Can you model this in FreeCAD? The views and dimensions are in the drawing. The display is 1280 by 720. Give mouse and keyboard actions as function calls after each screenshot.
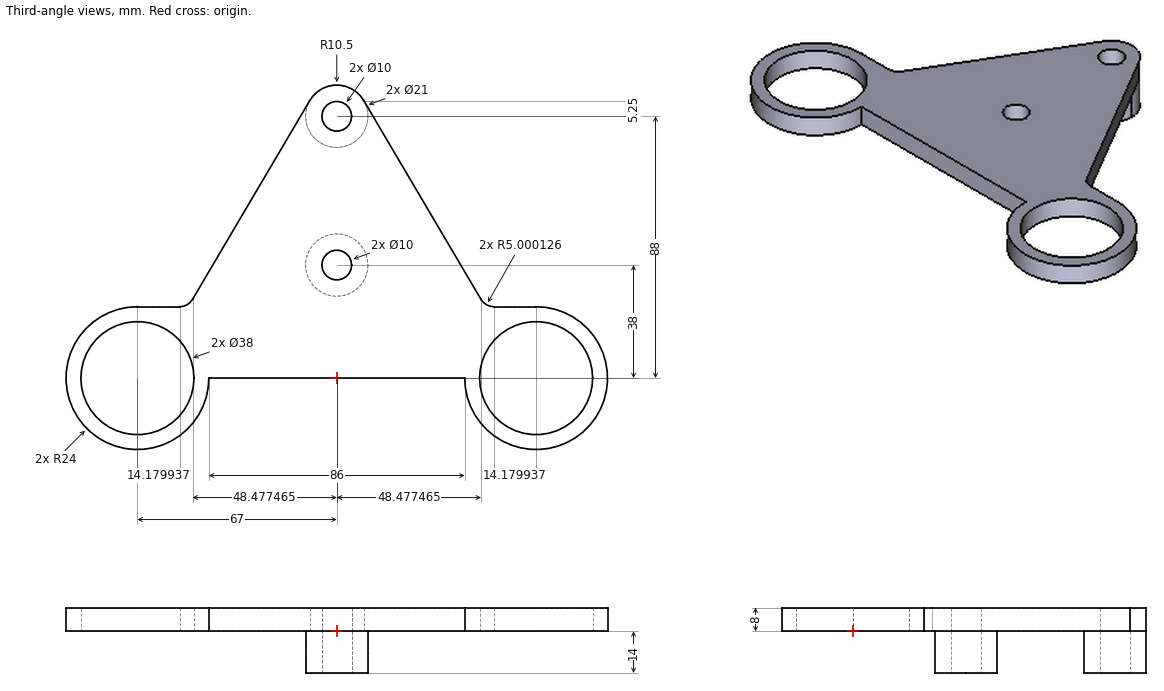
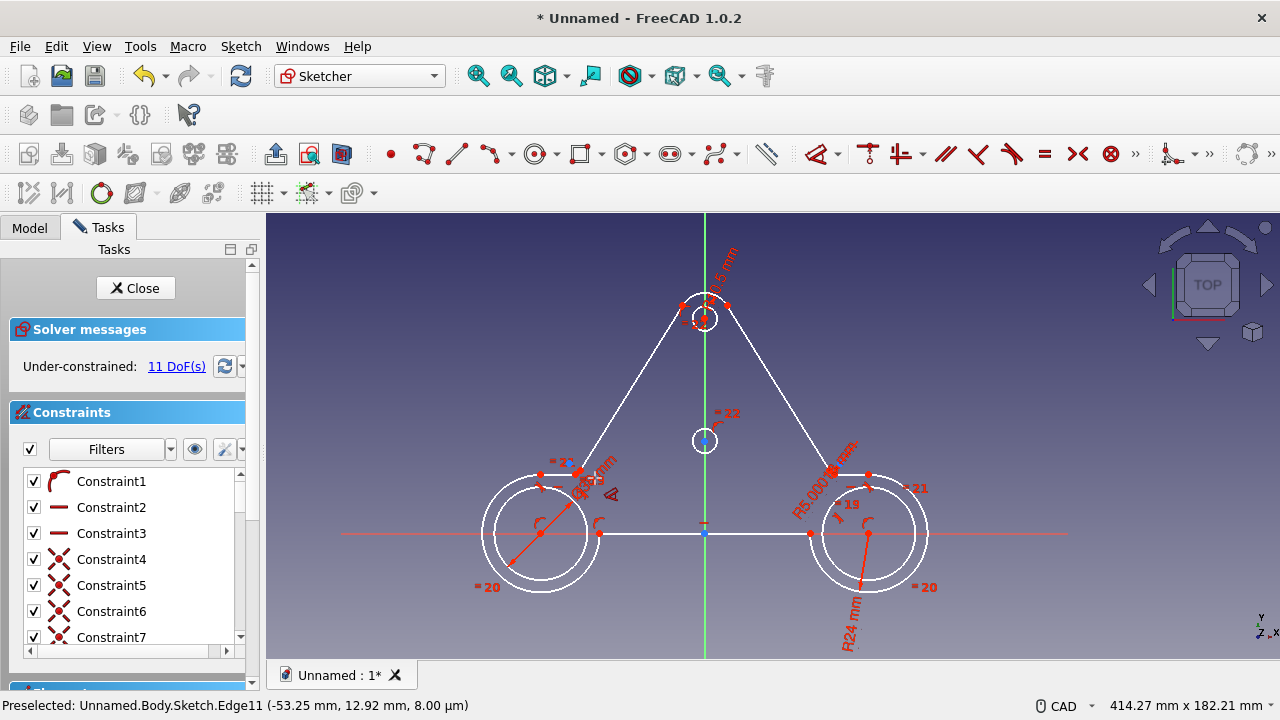
scroll(705, 429, up, 3)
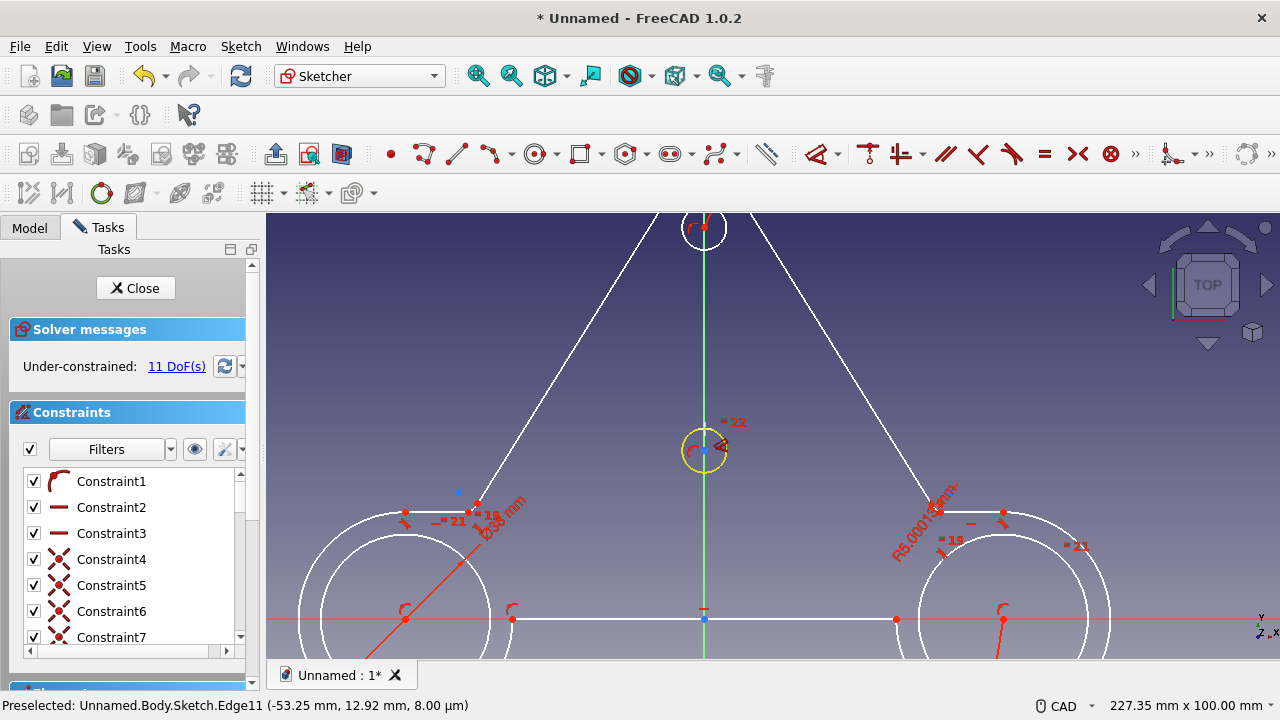
click(705, 428)
click(732, 403)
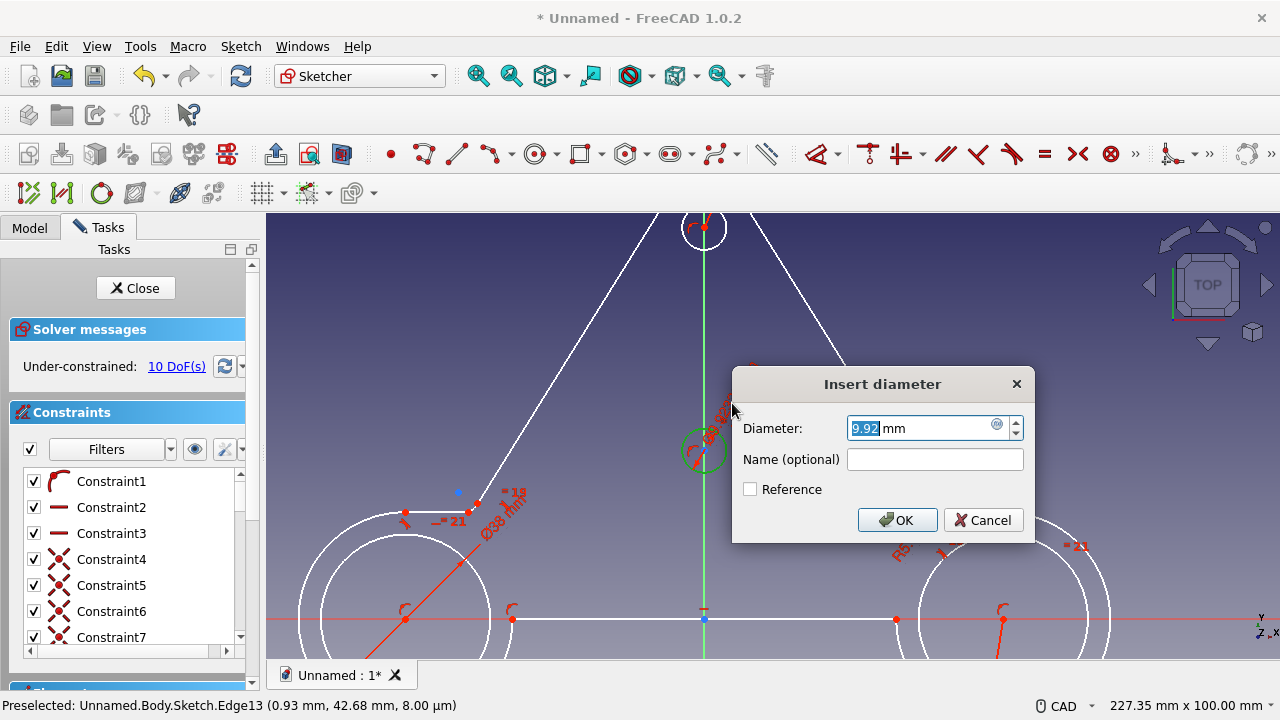
text(10)
key(Return)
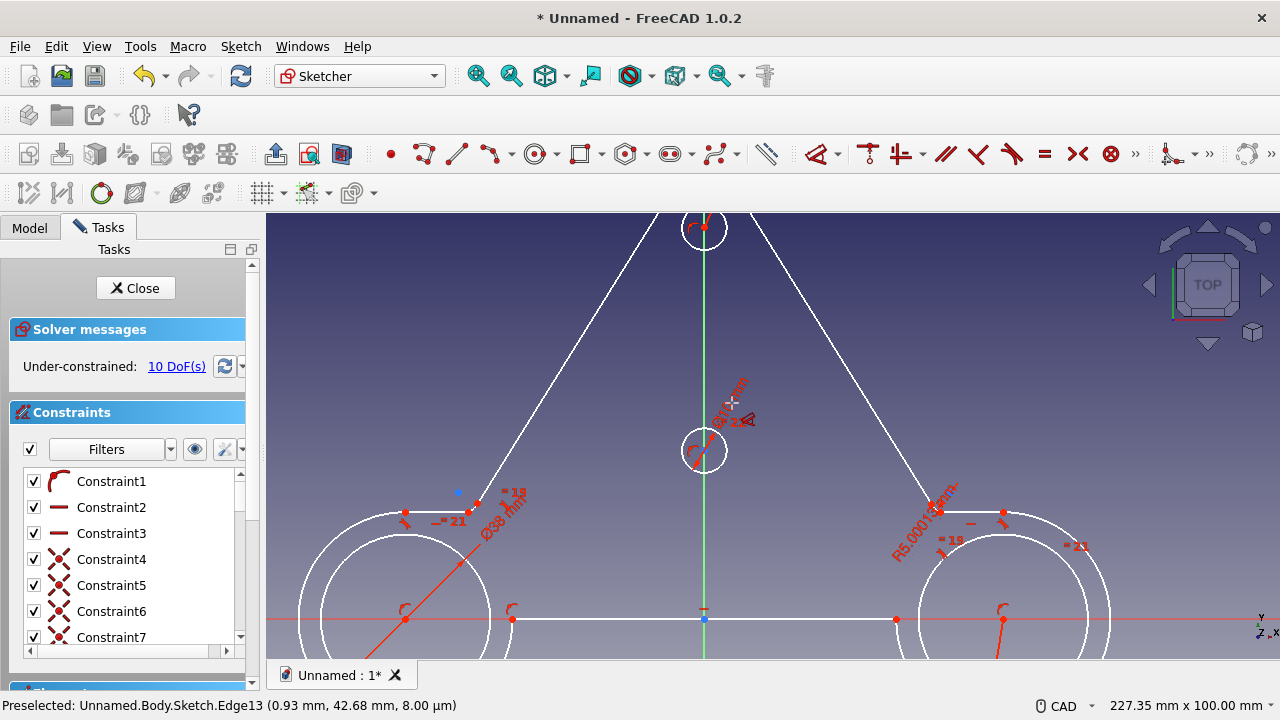
click(628, 619)
click(616, 585)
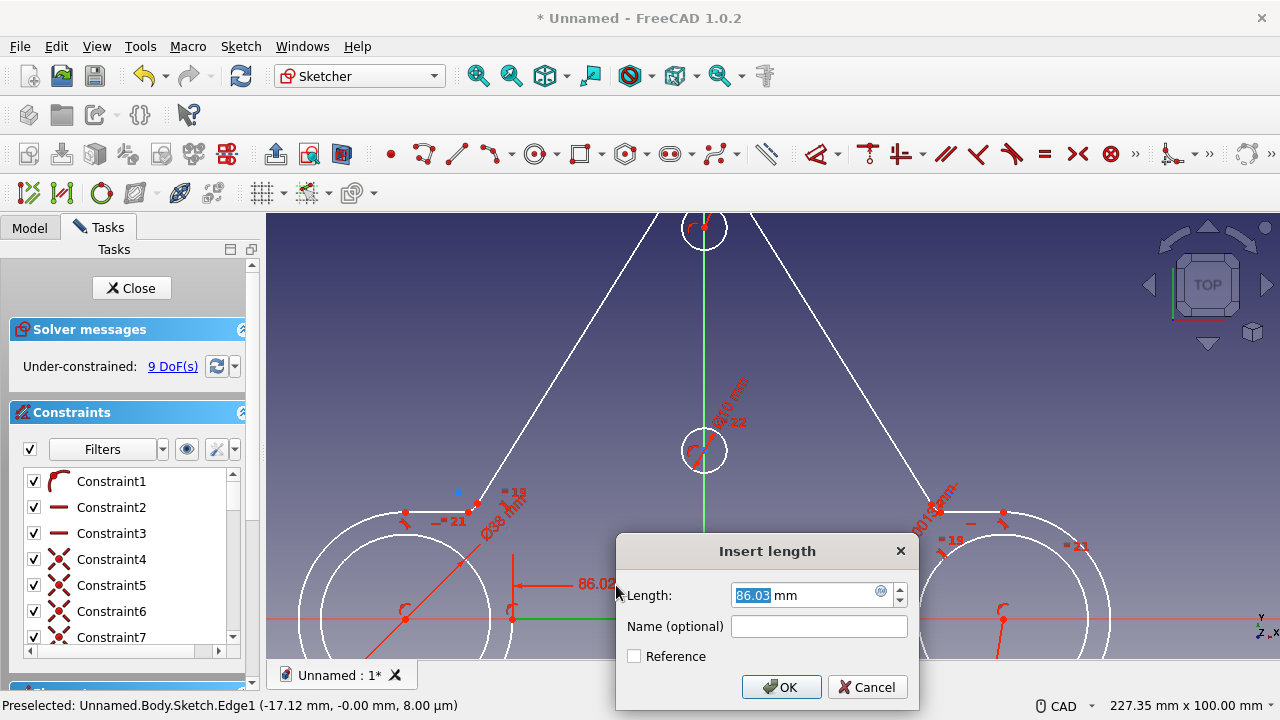
text(86)
key(Return)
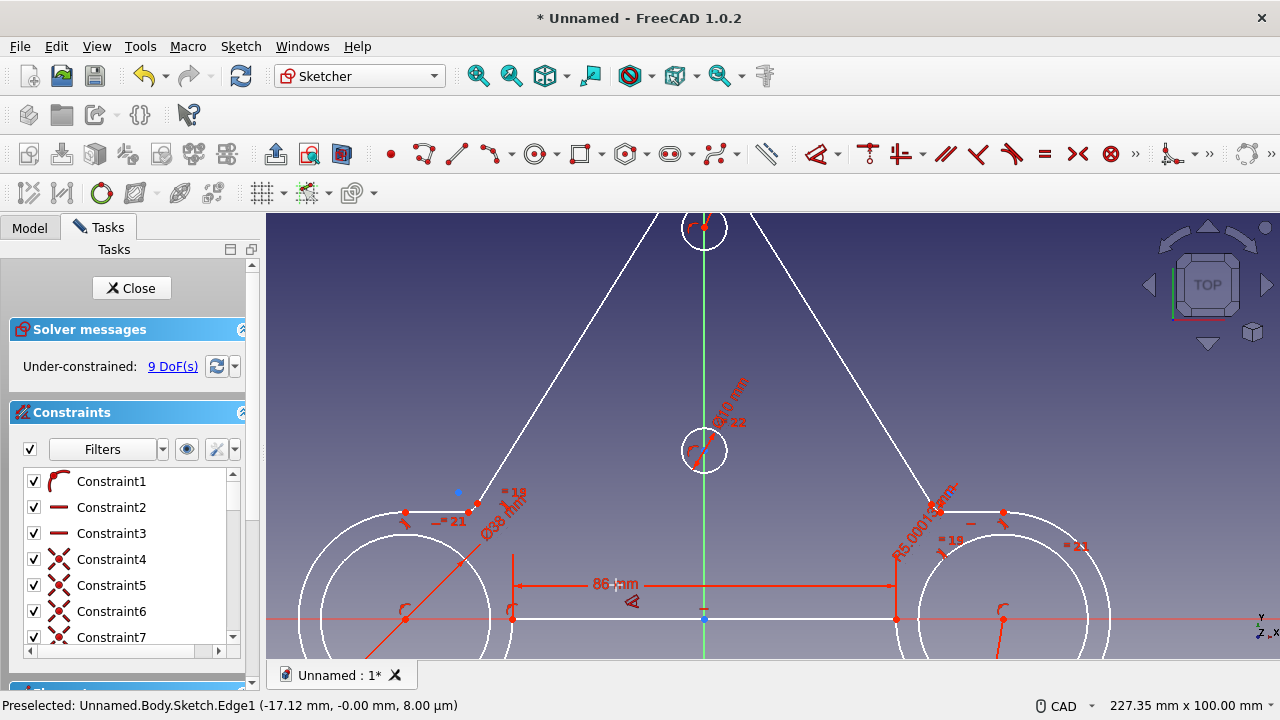
click(405, 619)
click(450, 585)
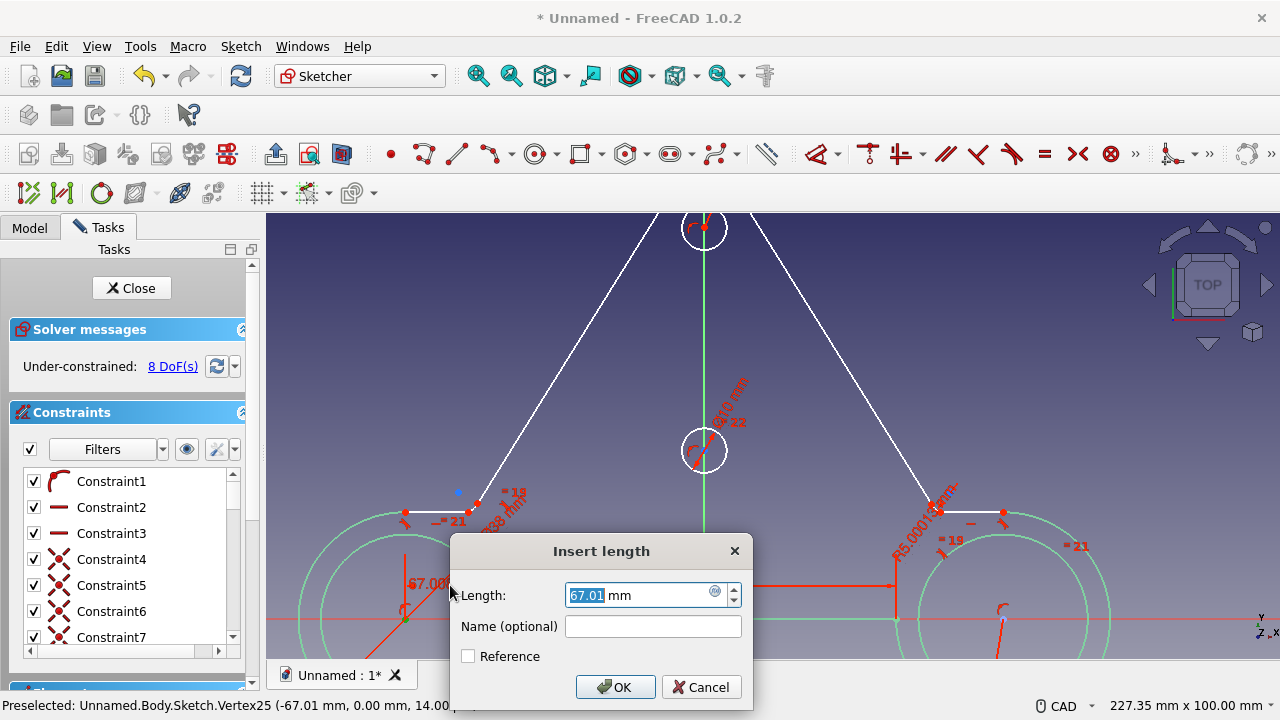
text(67)
key(Return)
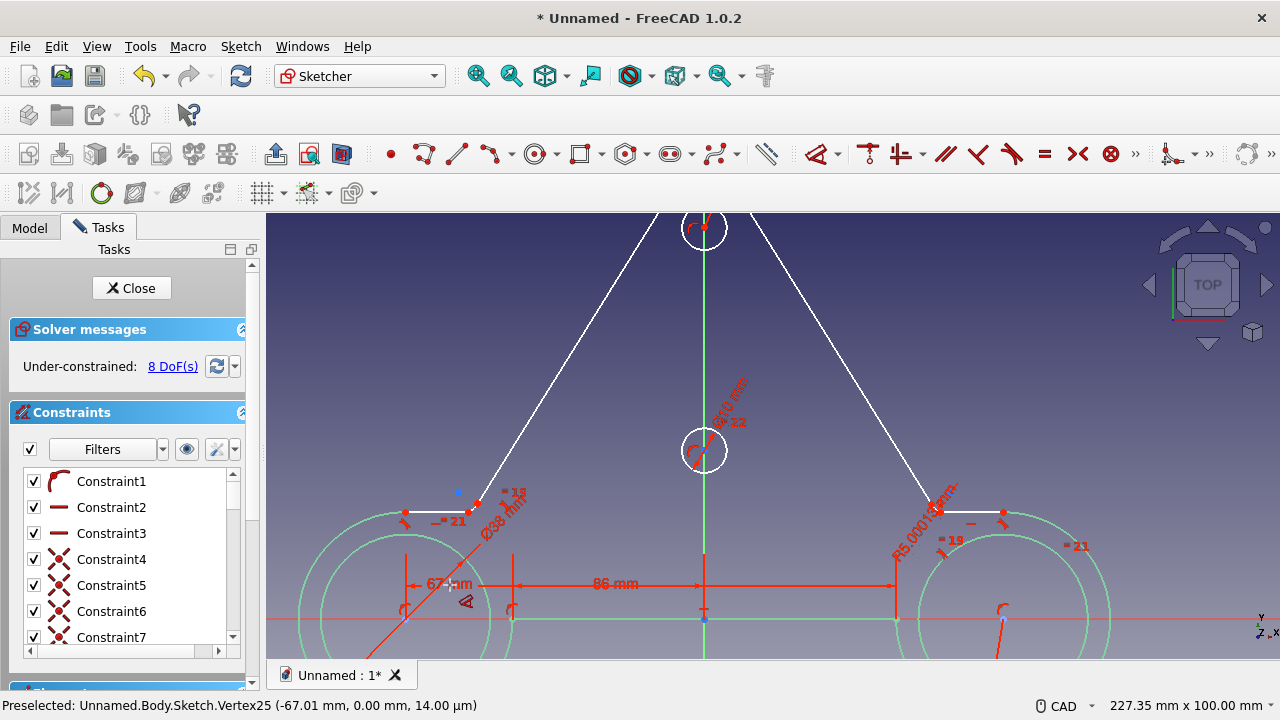
click(704, 451)
click(738, 535)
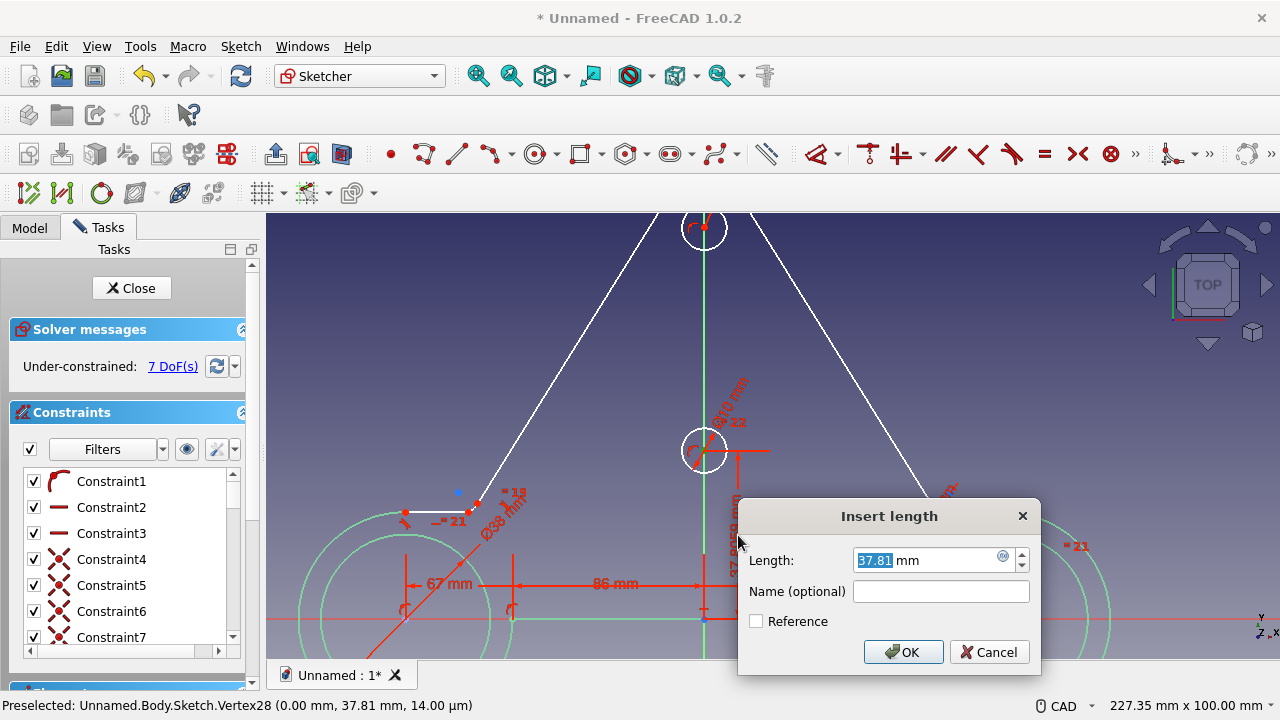
text(38)
key(Return)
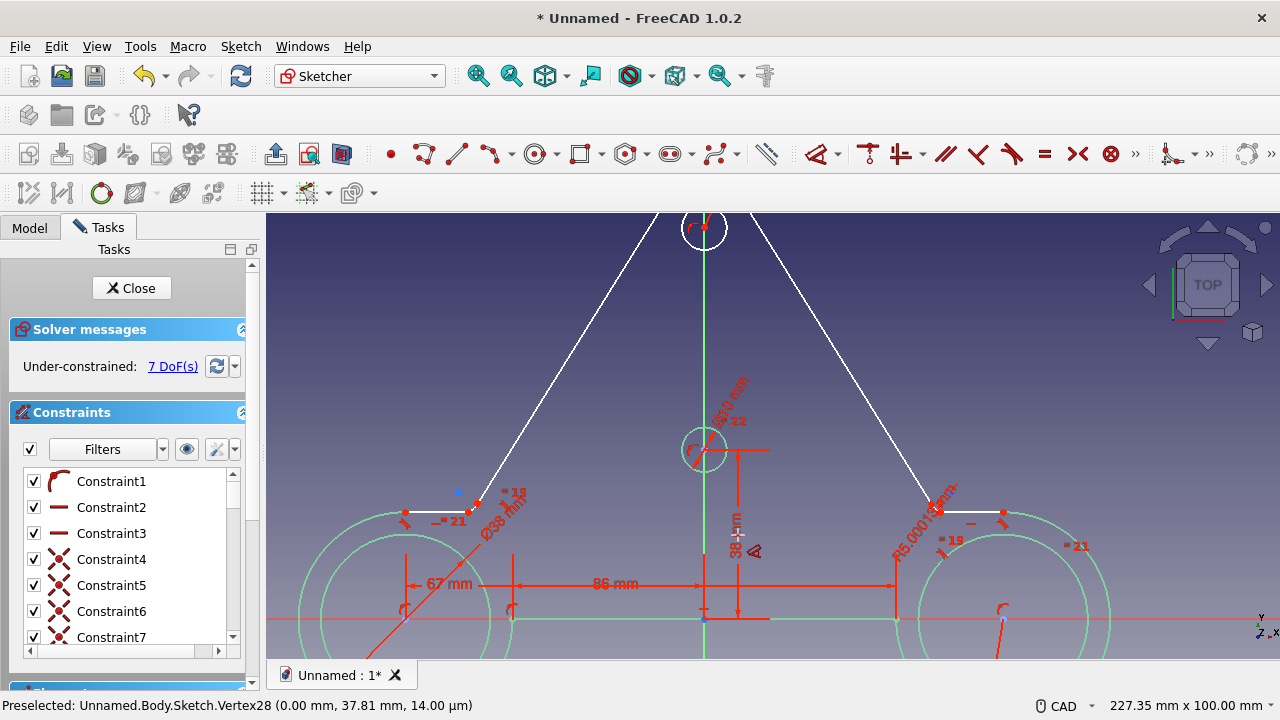
scroll(705, 429, down, 3)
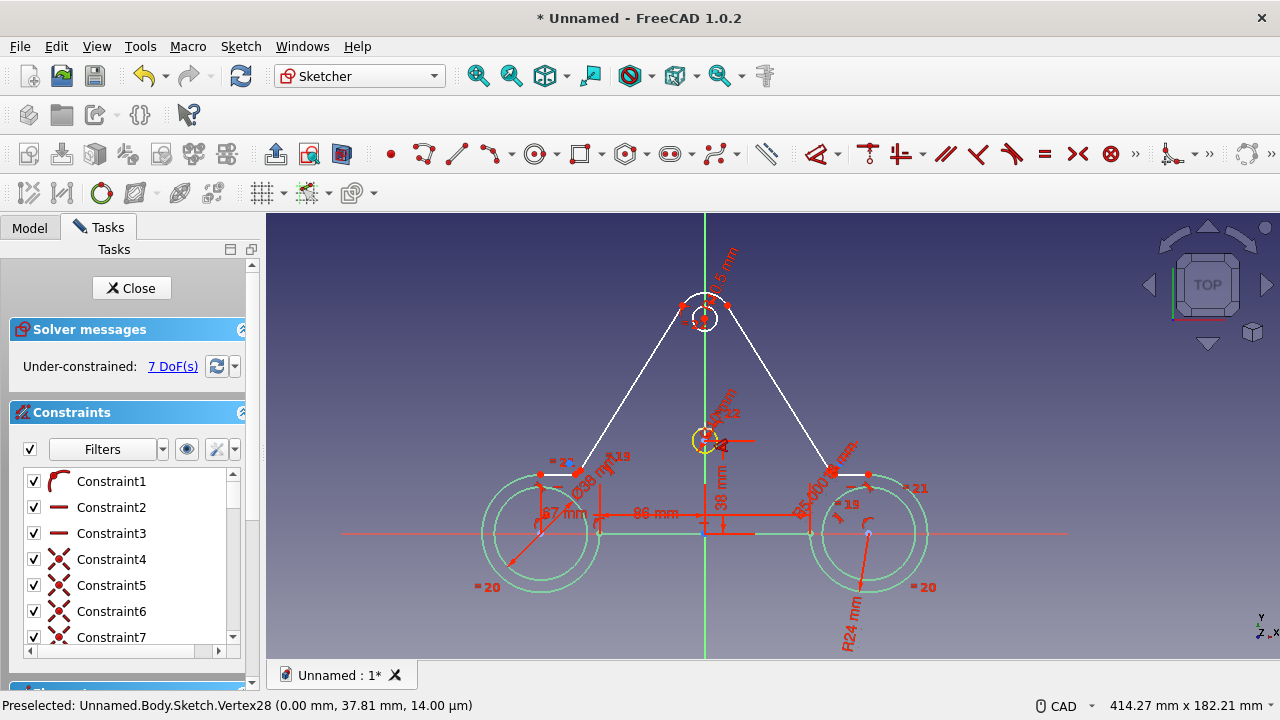
click(705, 319)
click(739, 377)